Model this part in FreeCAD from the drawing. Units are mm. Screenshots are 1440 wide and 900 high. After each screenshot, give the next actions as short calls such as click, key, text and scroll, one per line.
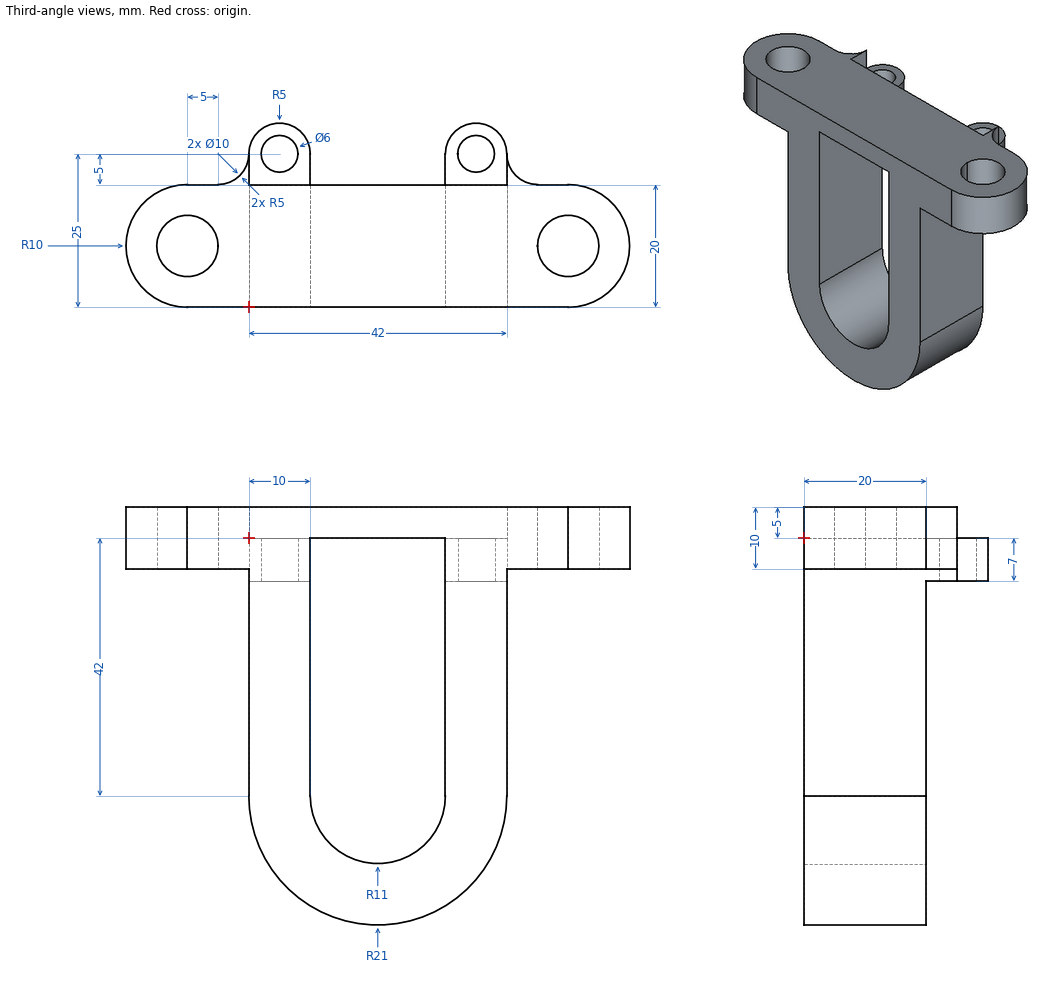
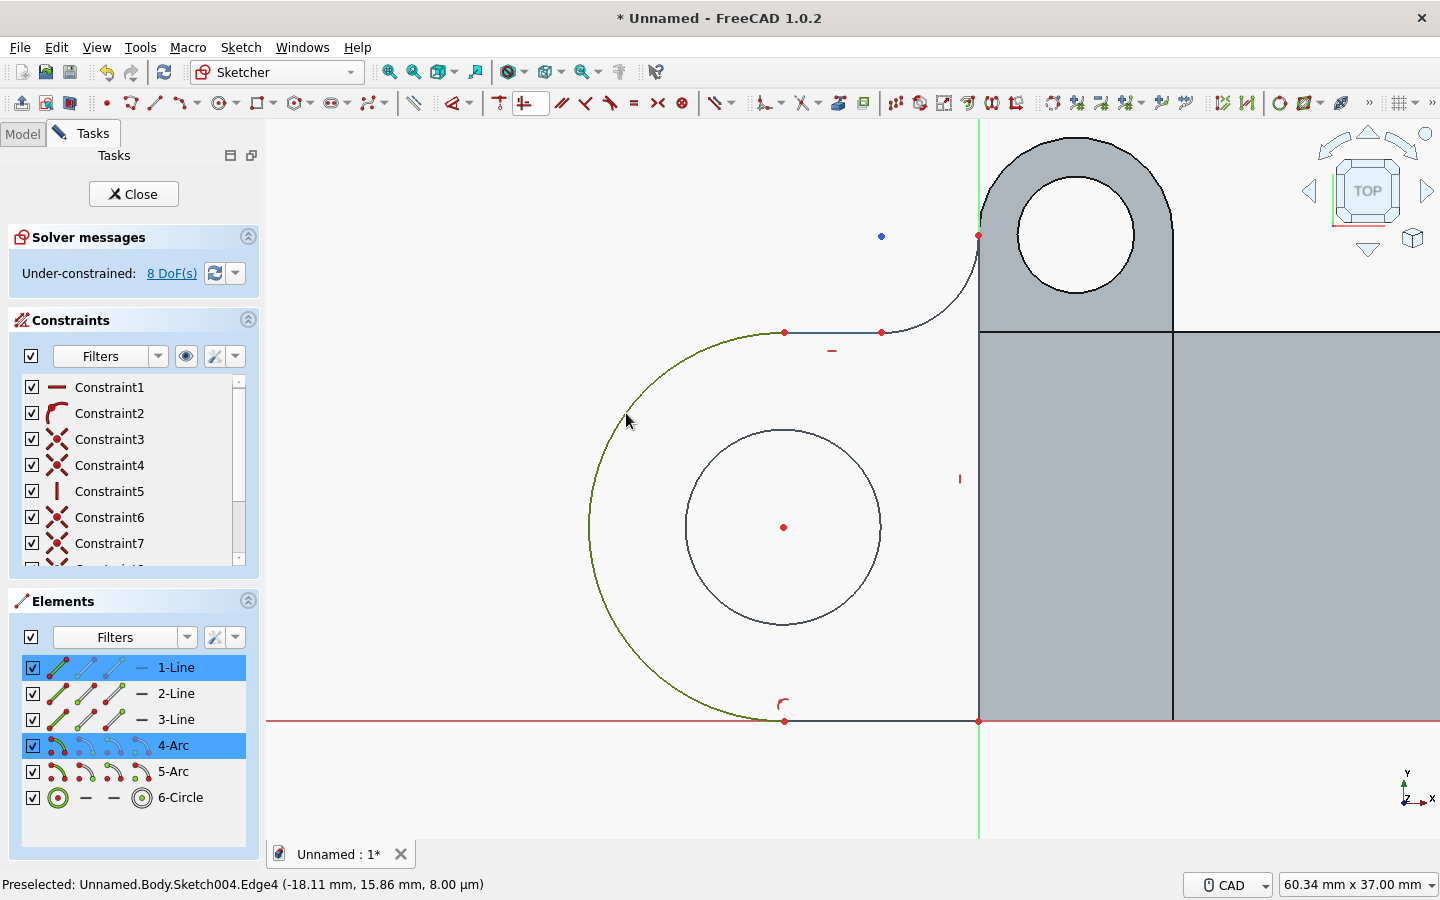
click(610, 104)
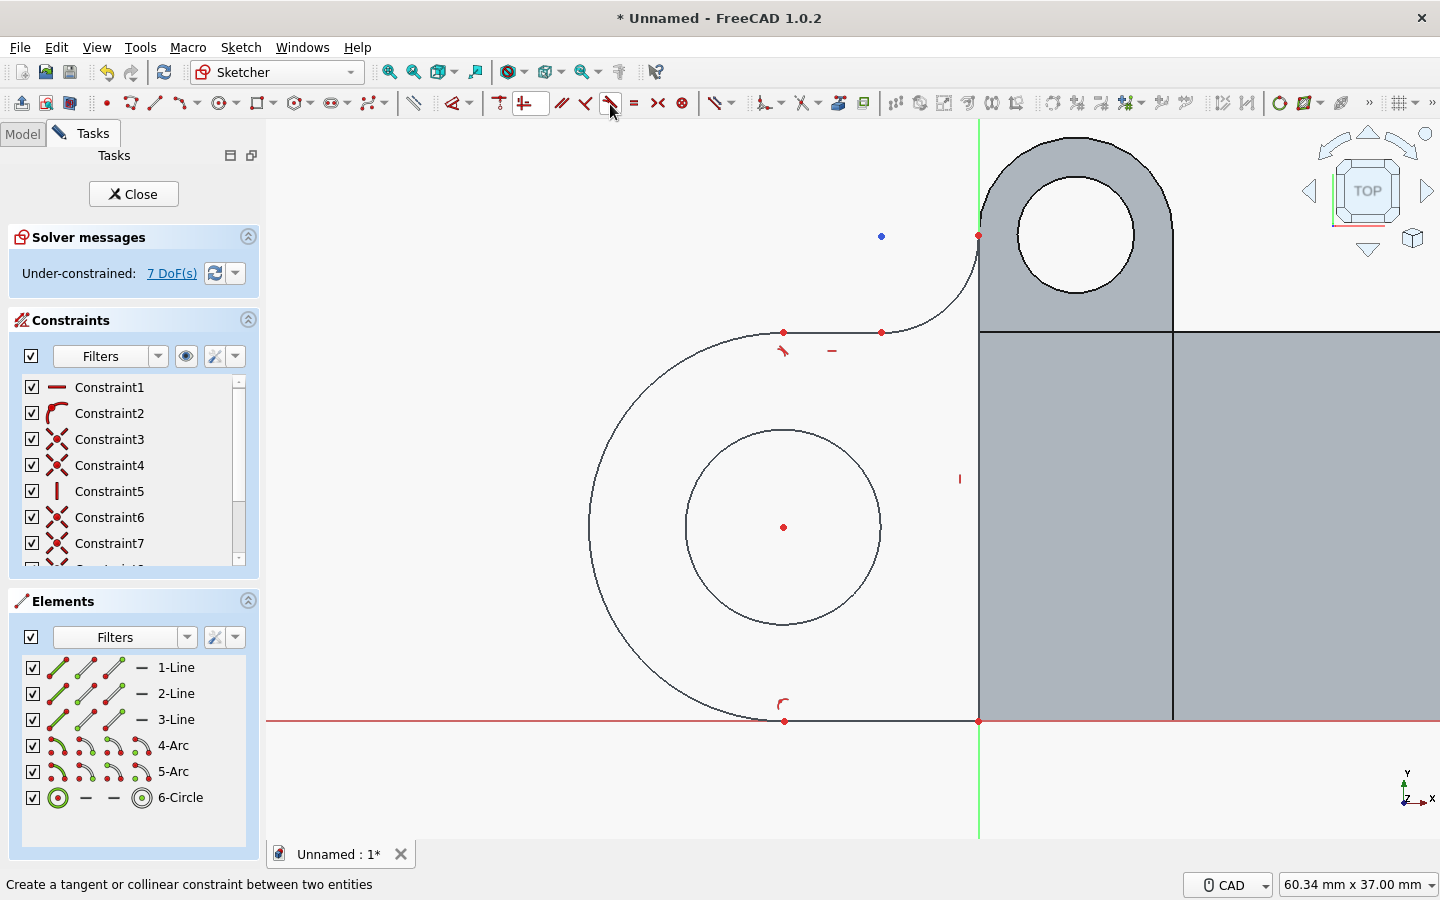
click(852, 333)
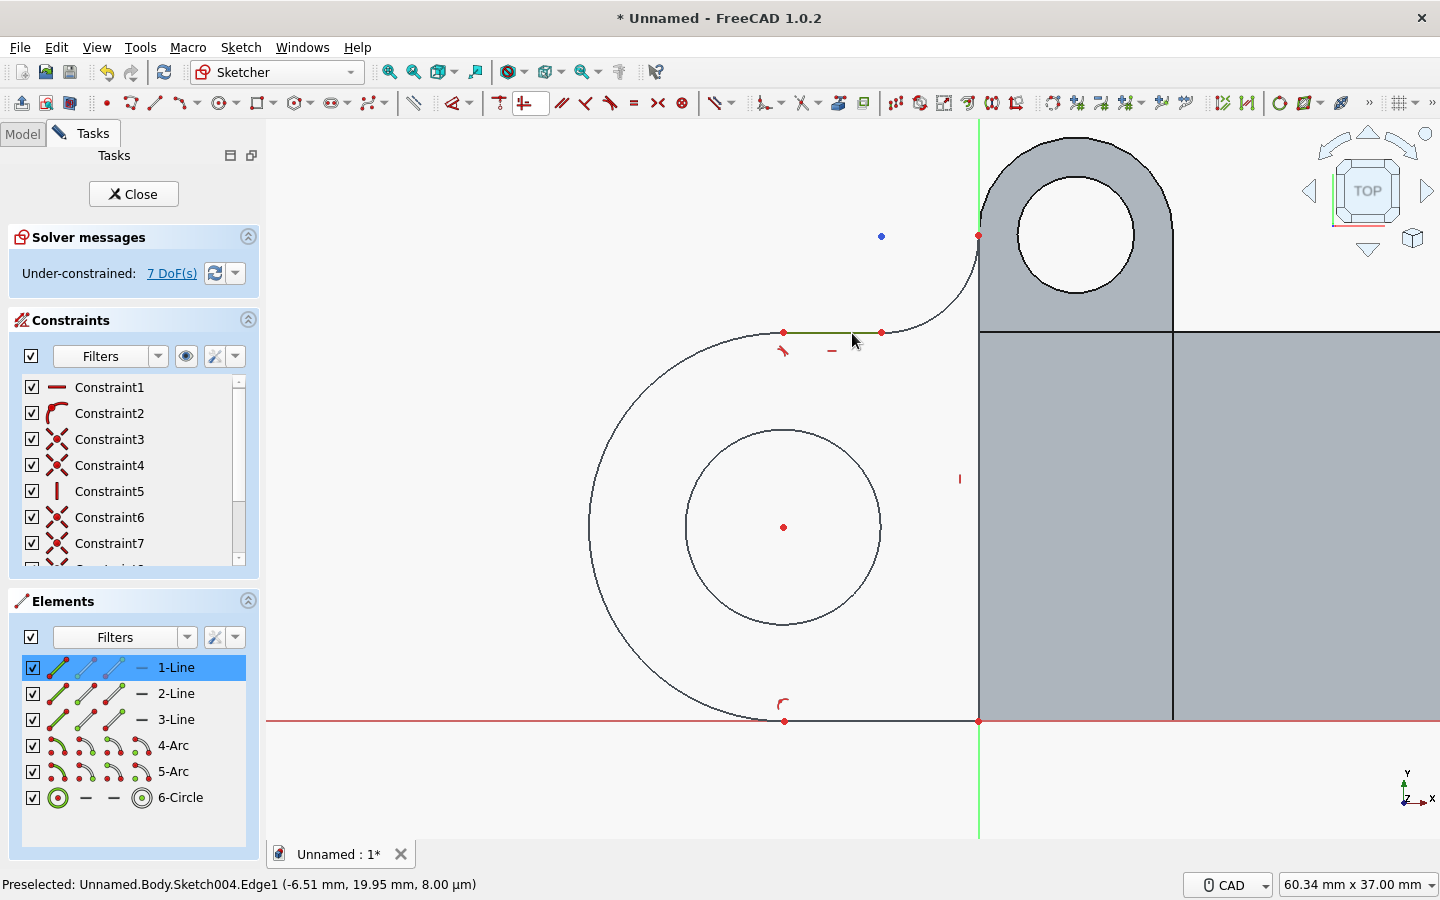
click(925, 323)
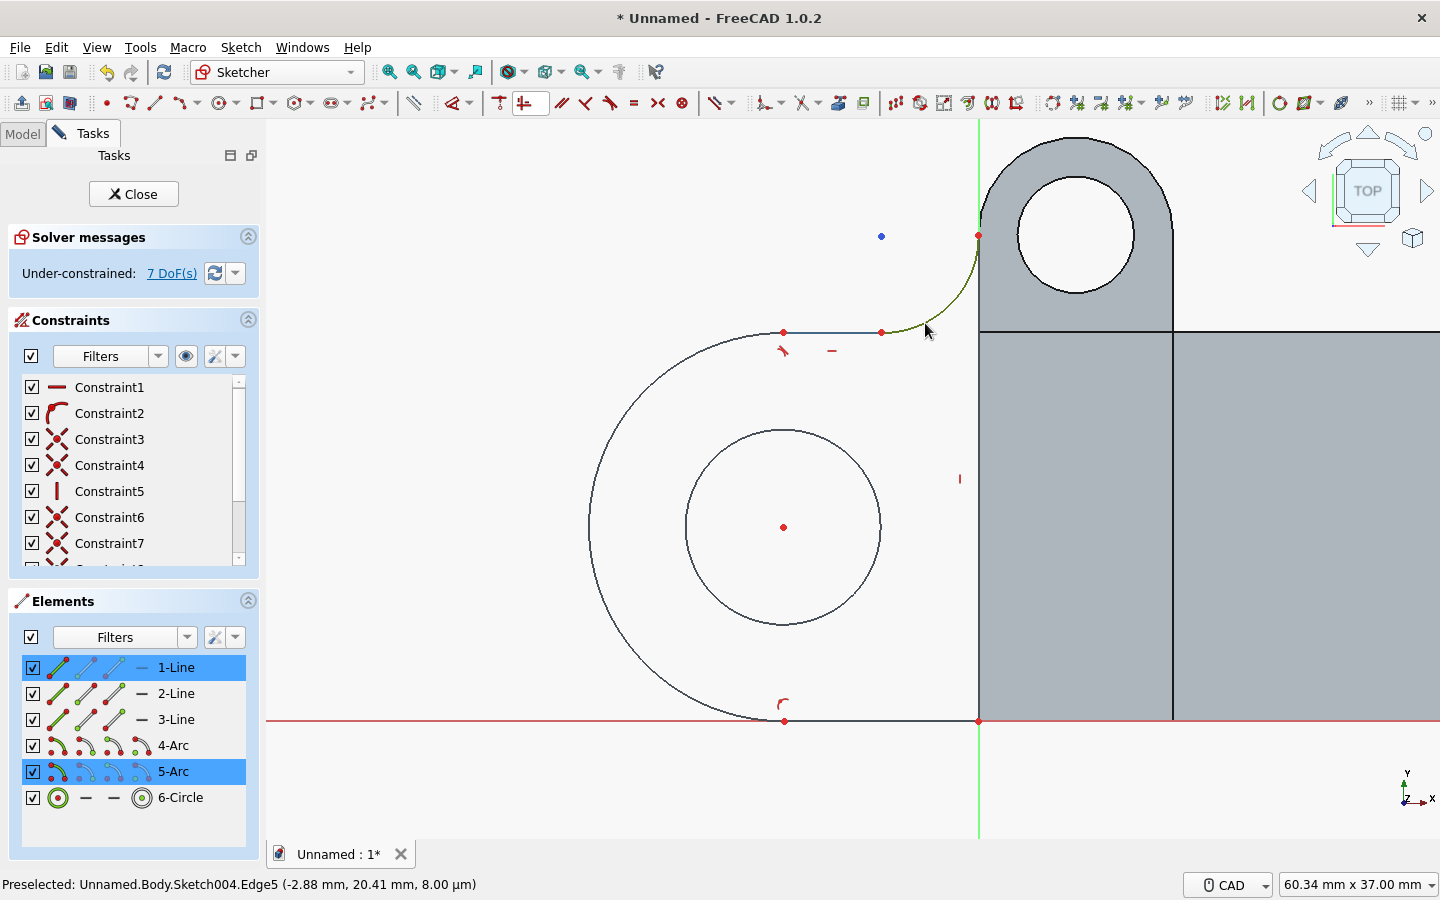
click(610, 104)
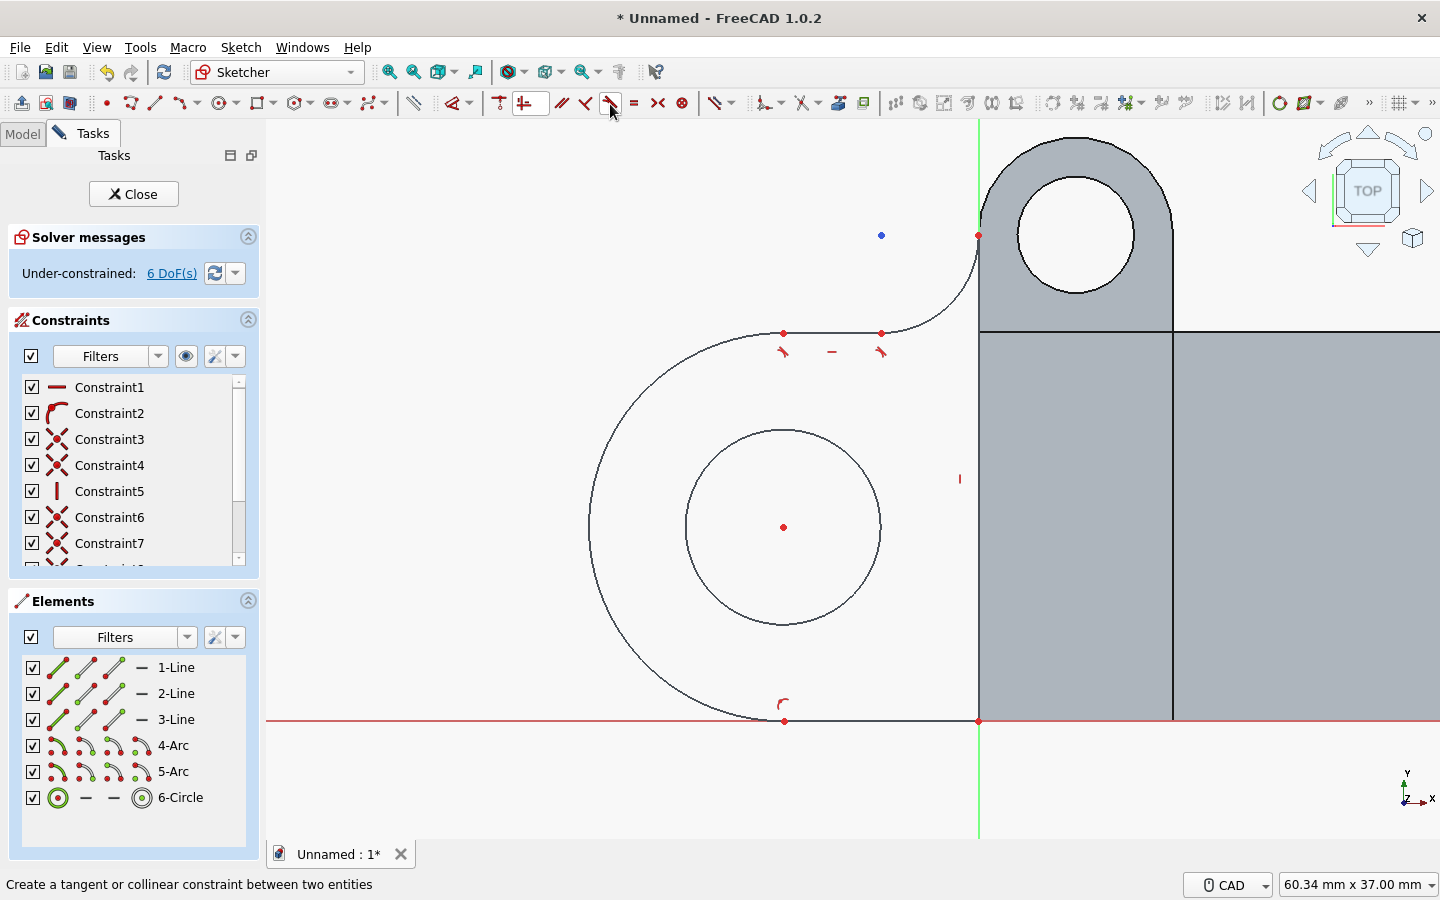
click(842, 721)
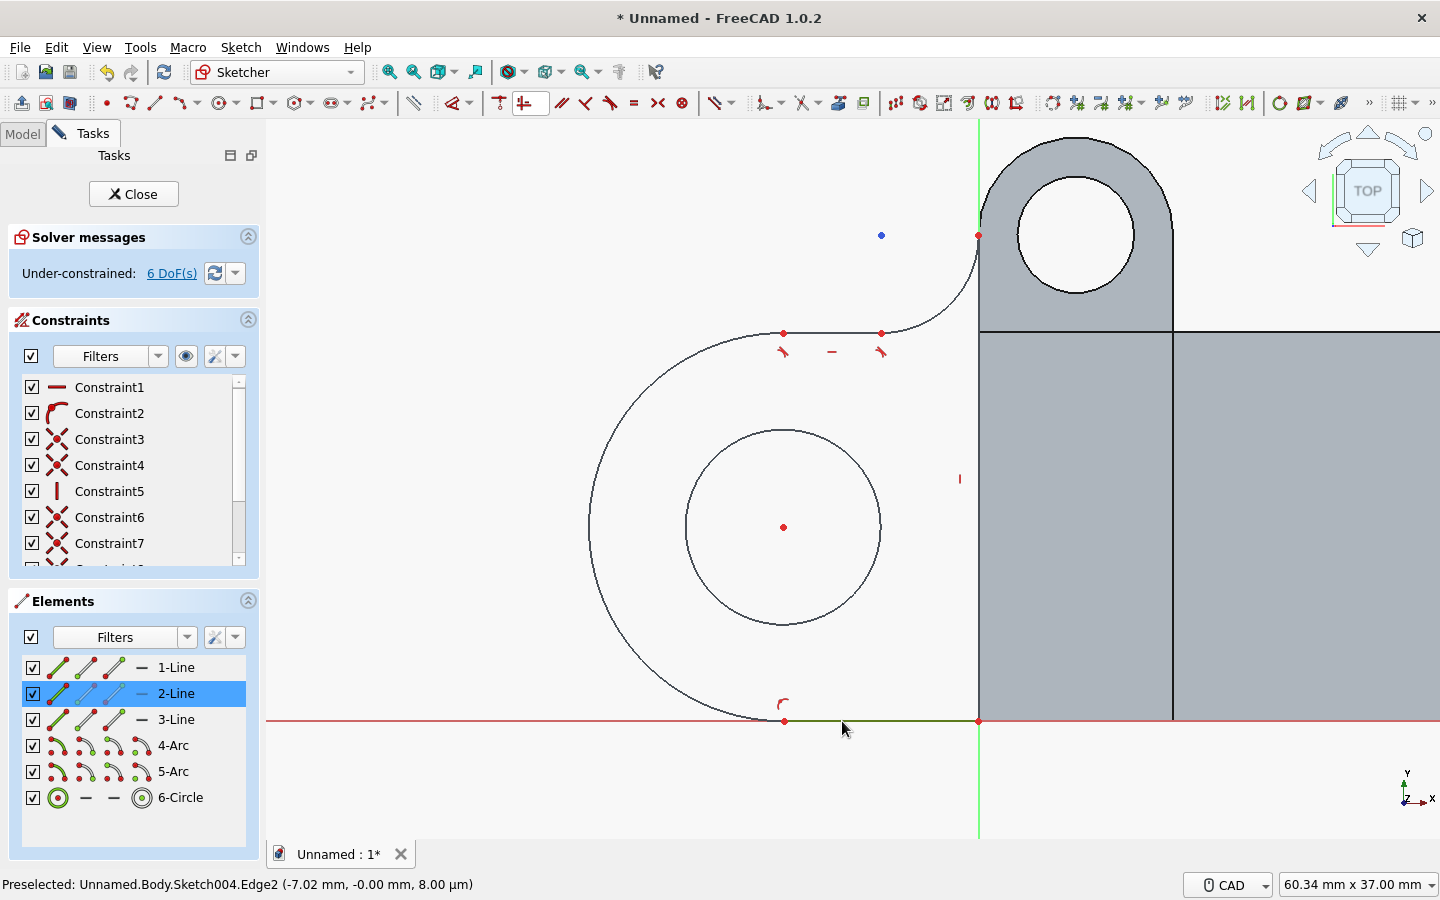
click(626, 413)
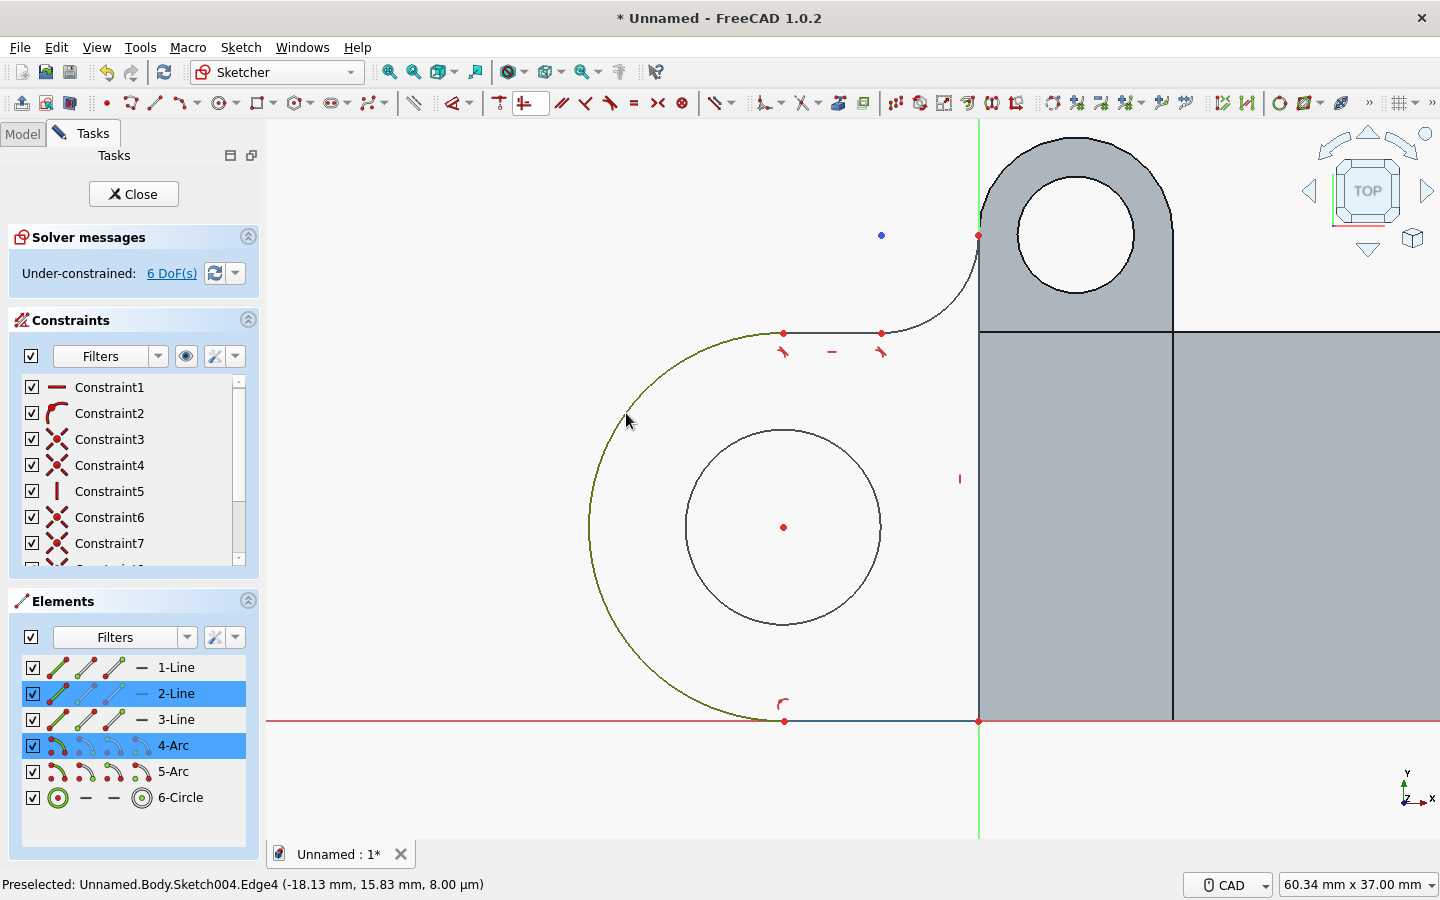
click(610, 104)